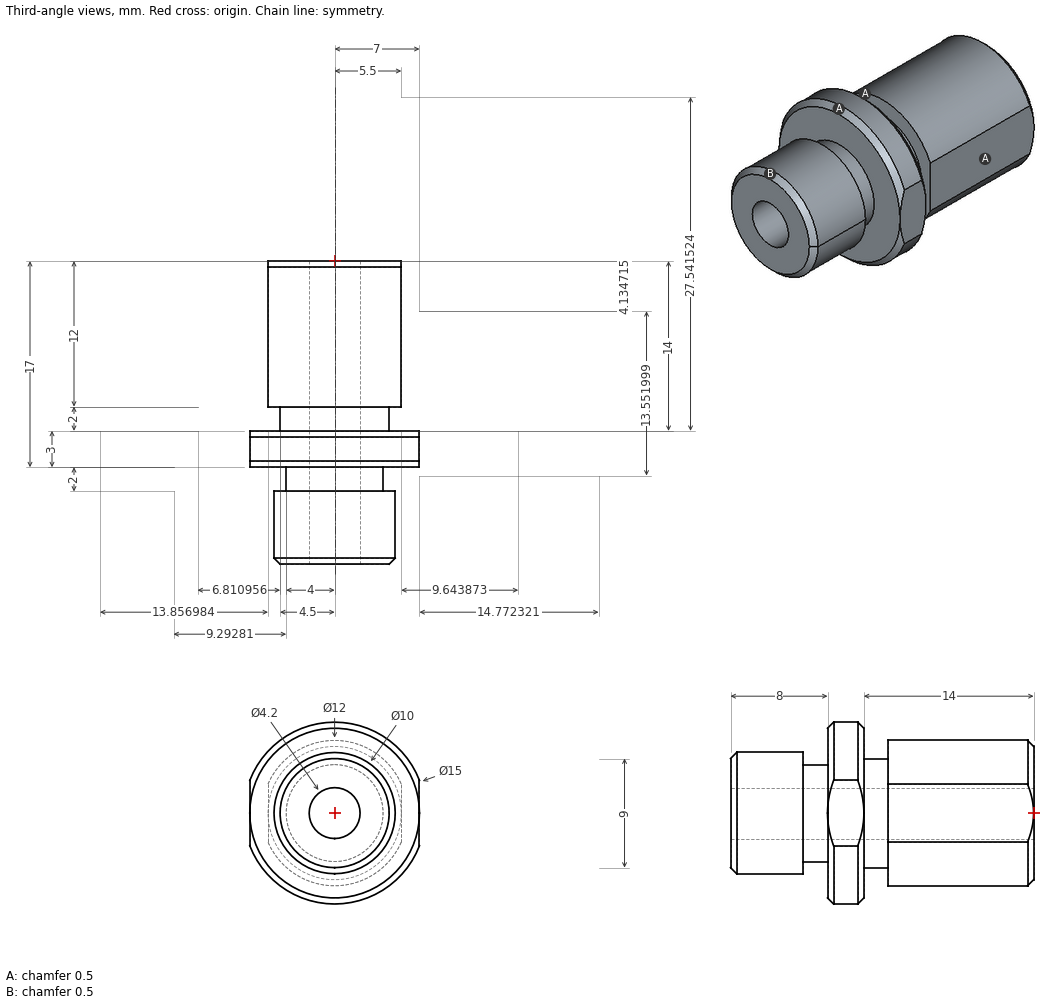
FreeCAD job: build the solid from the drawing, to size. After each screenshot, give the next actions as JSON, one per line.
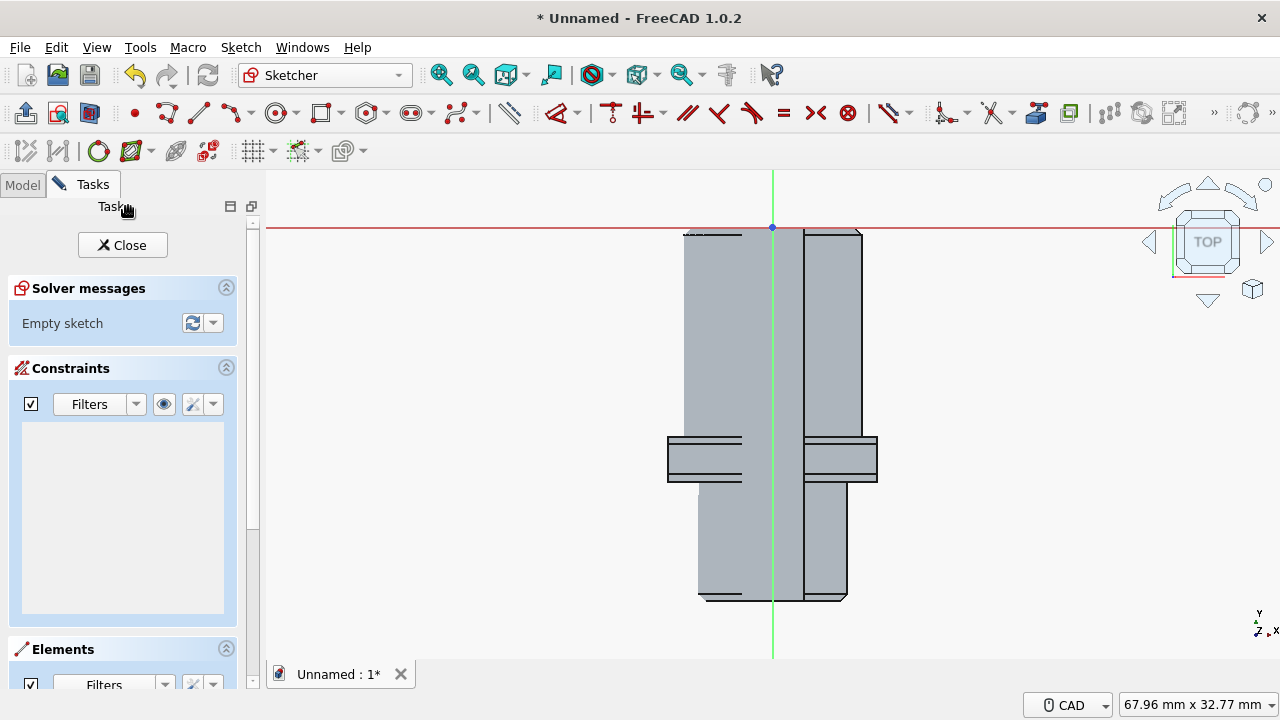
{"action": "scroll", "coordinate": [629, 631], "scroll_direction": "down", "scroll_amount": 2}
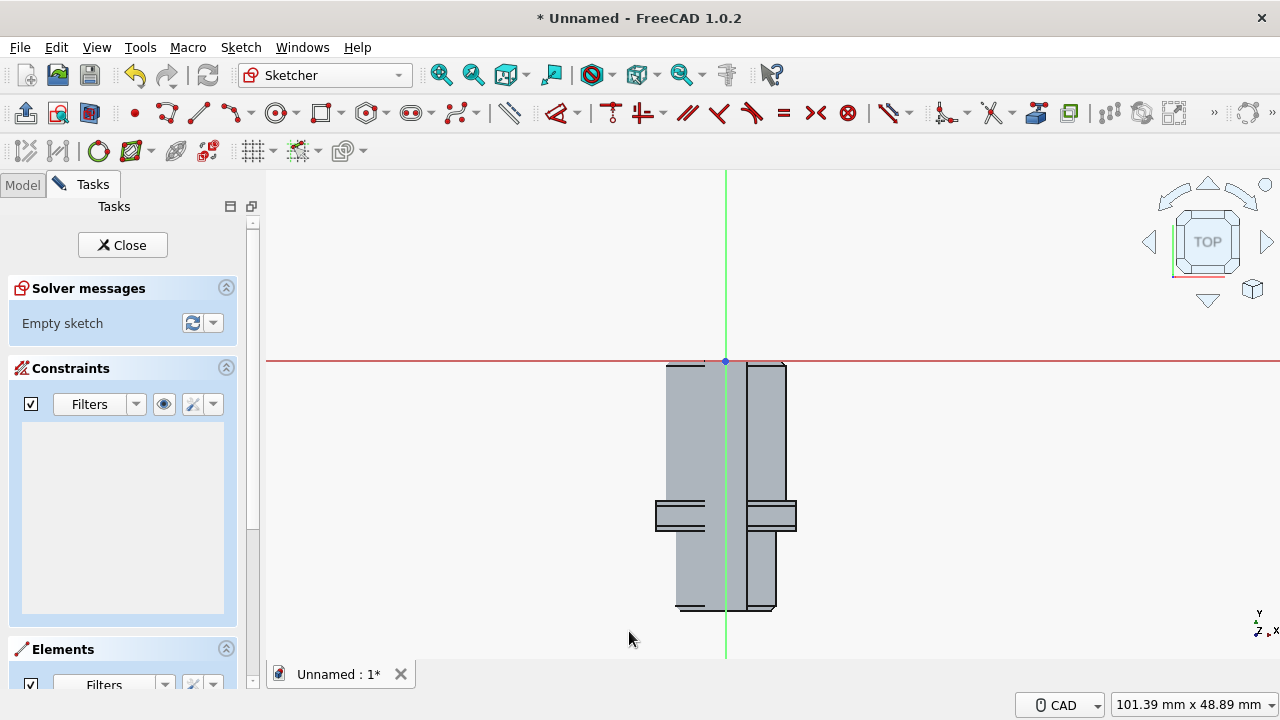
{"action": "key", "text": "g r"}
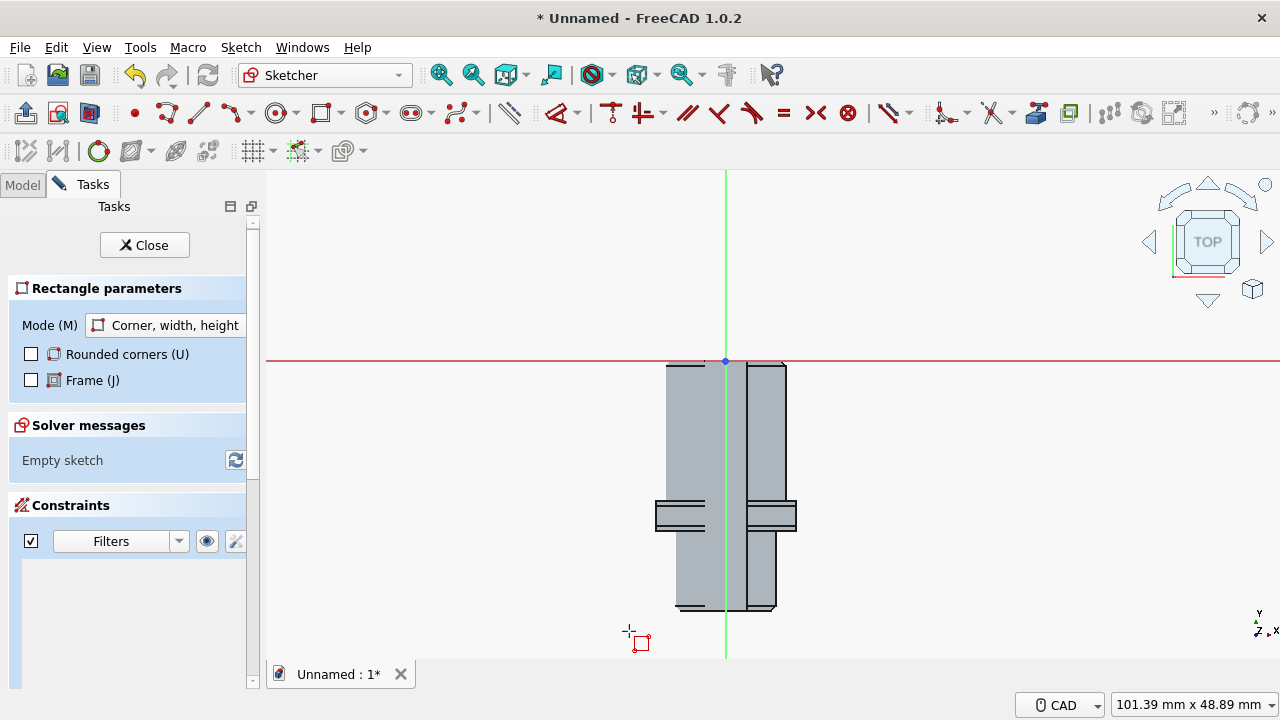
{"action": "left_click", "coordinate": [781, 226]}
{"action": "left_click", "coordinate": [877, 501]}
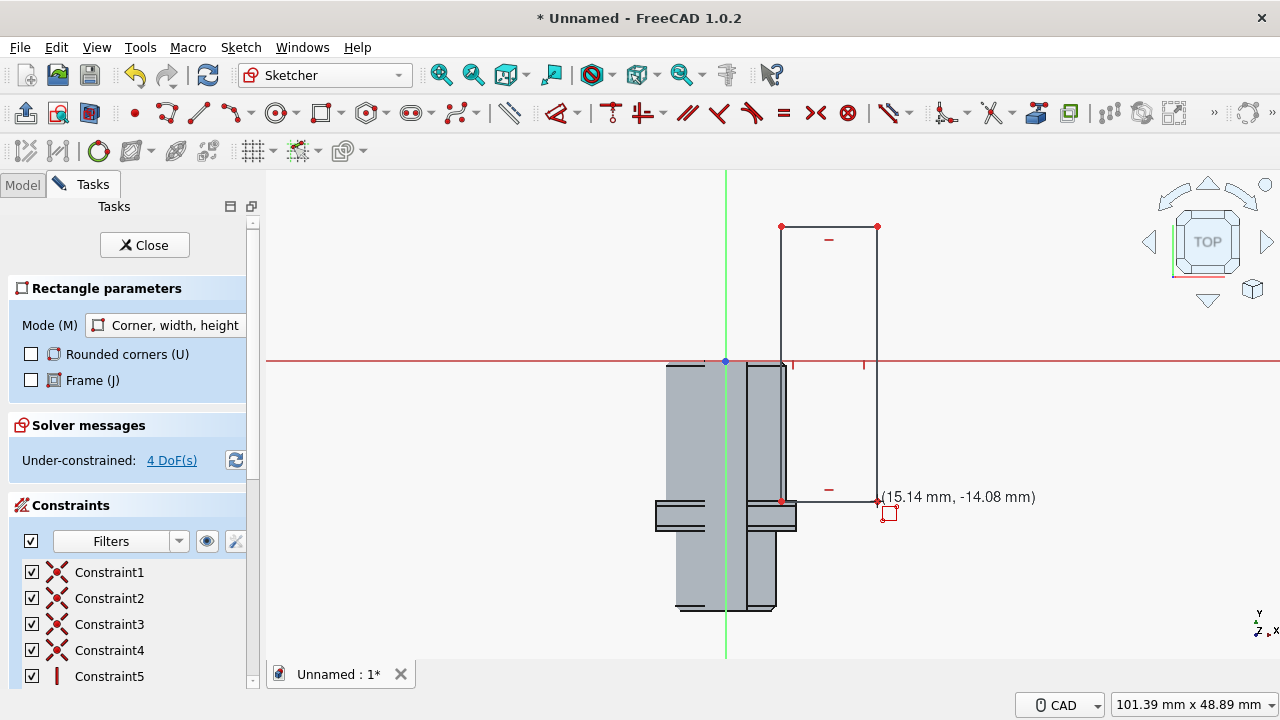
{"action": "left_click", "coordinate": [532, 226]}
{"action": "left_click", "coordinate": [671, 501]}
{"action": "key", "text": "Escape"}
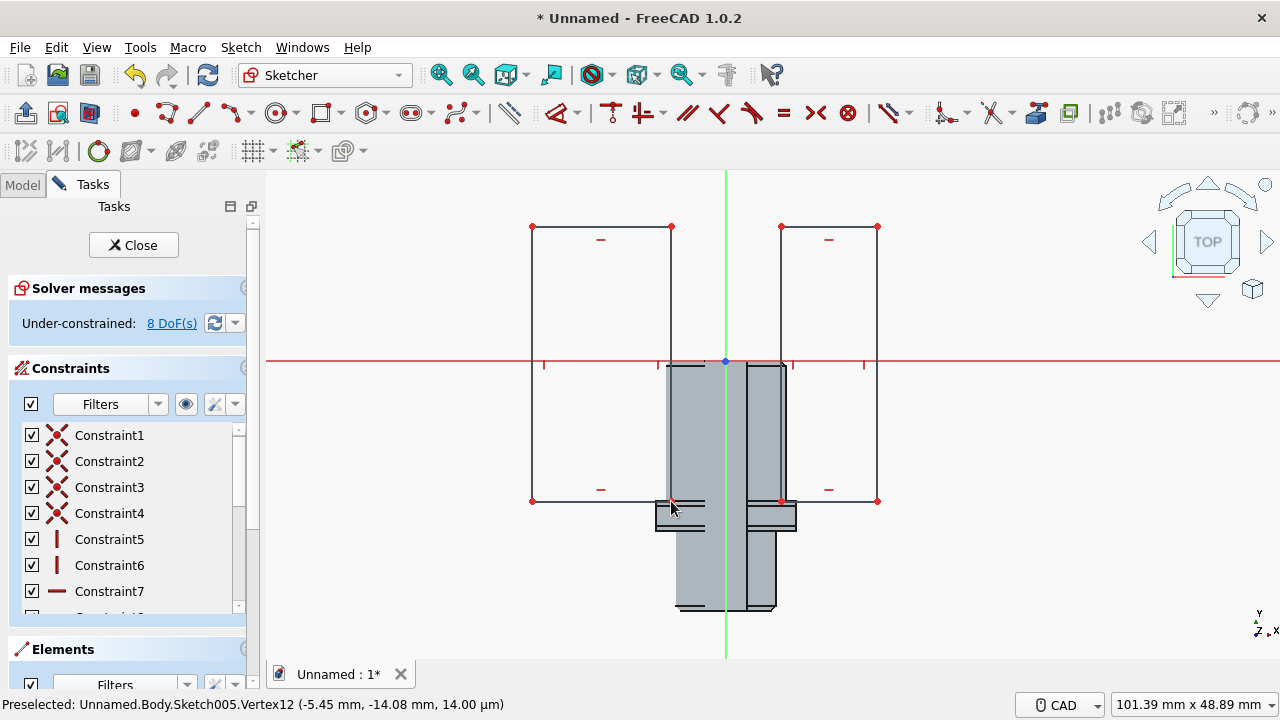
{"action": "left_click", "coordinate": [781, 502]}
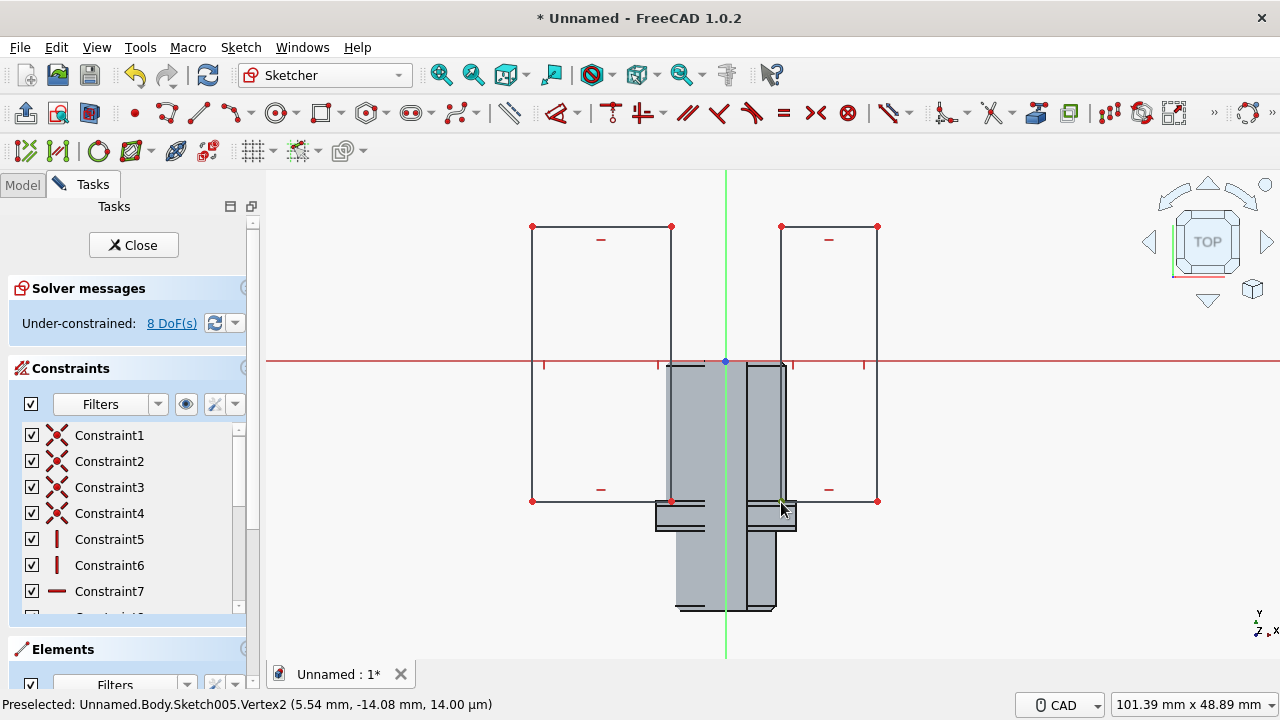
{"action": "left_click", "coordinate": [671, 502]}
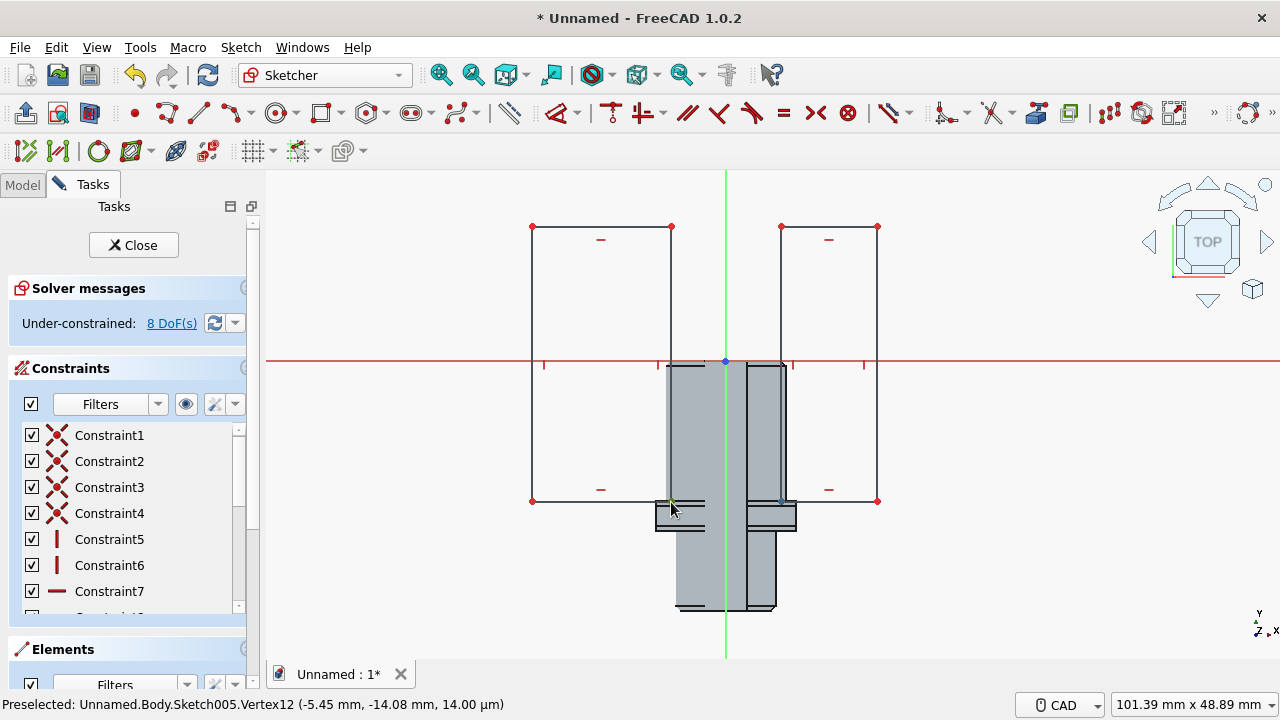
{"action": "left_click", "coordinate": [726, 600]}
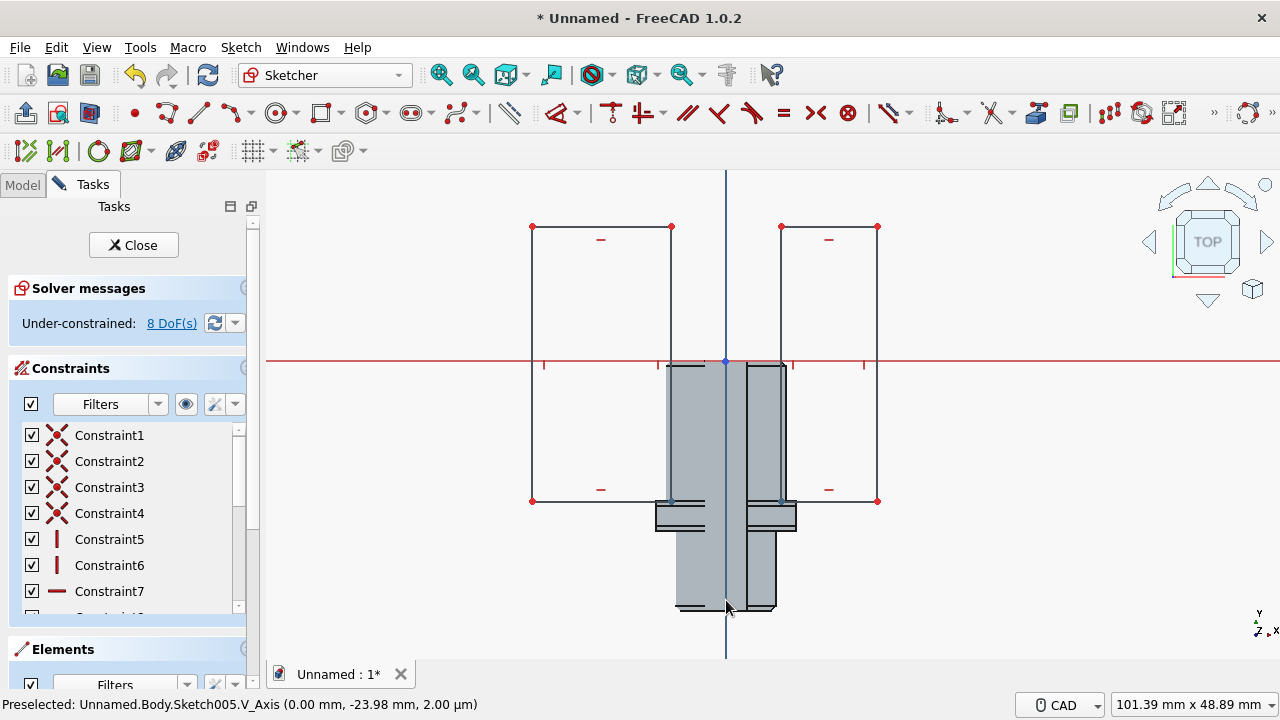
{"action": "key", "text": "s"}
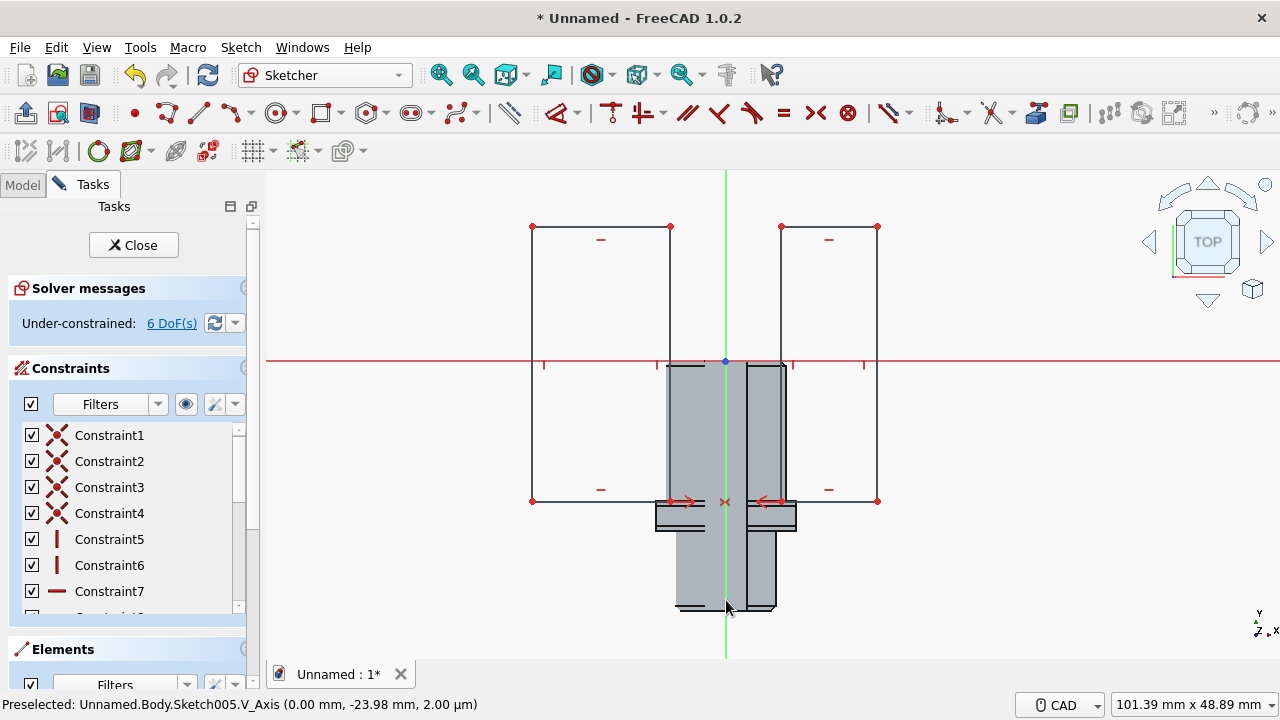
{"action": "key", "text": "d"}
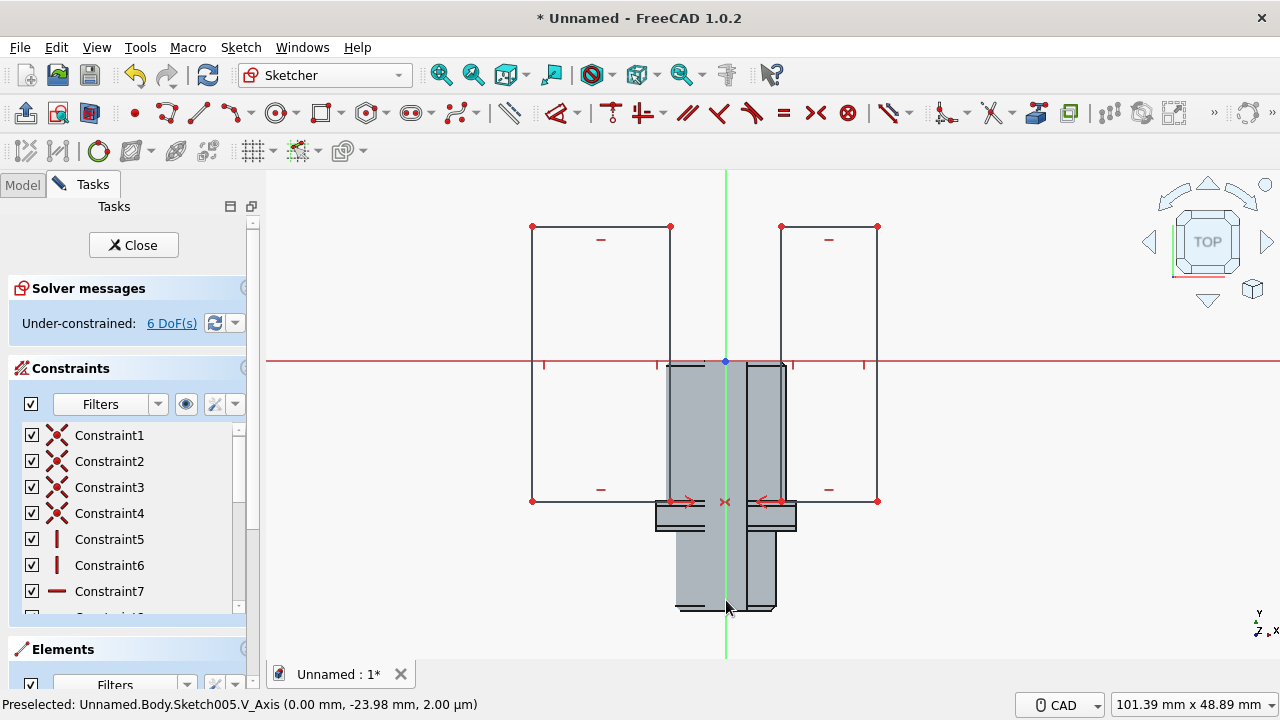
{"action": "left_click", "coordinate": [781, 502]}
{"action": "left_click", "coordinate": [815, 432]}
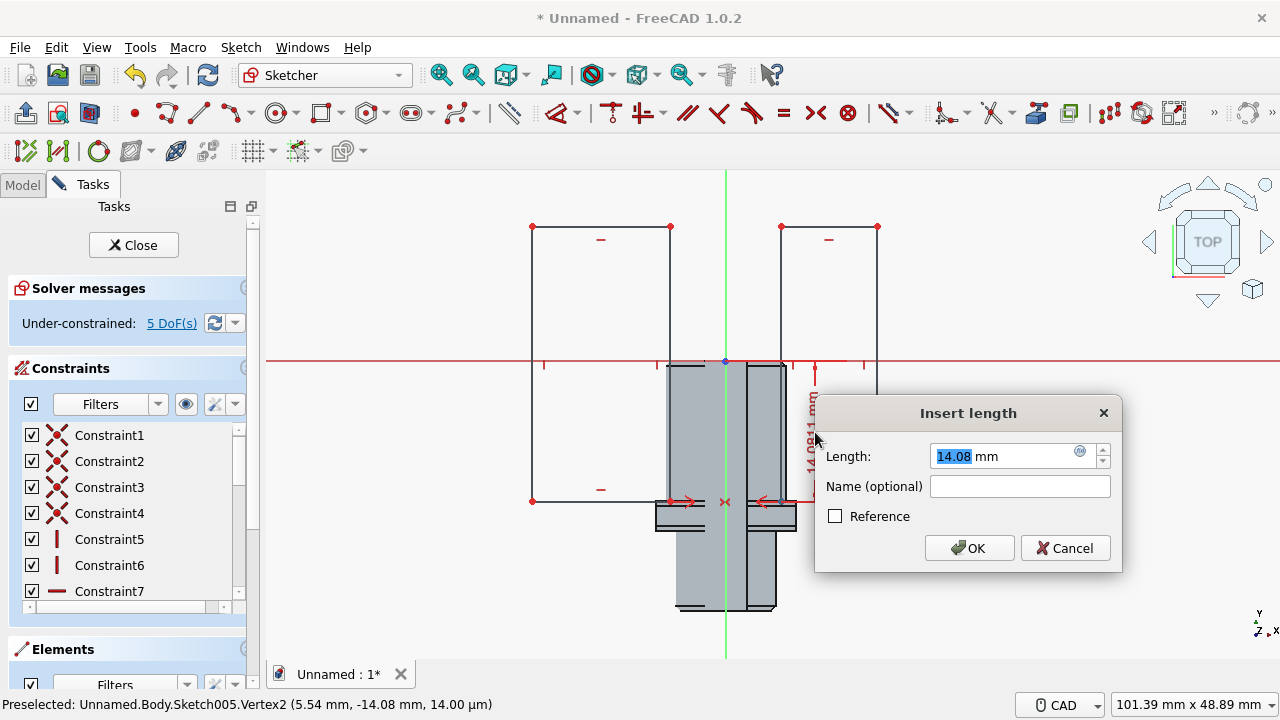
{"action": "type", "text": "14"}
{"action": "key", "text": "Return"}